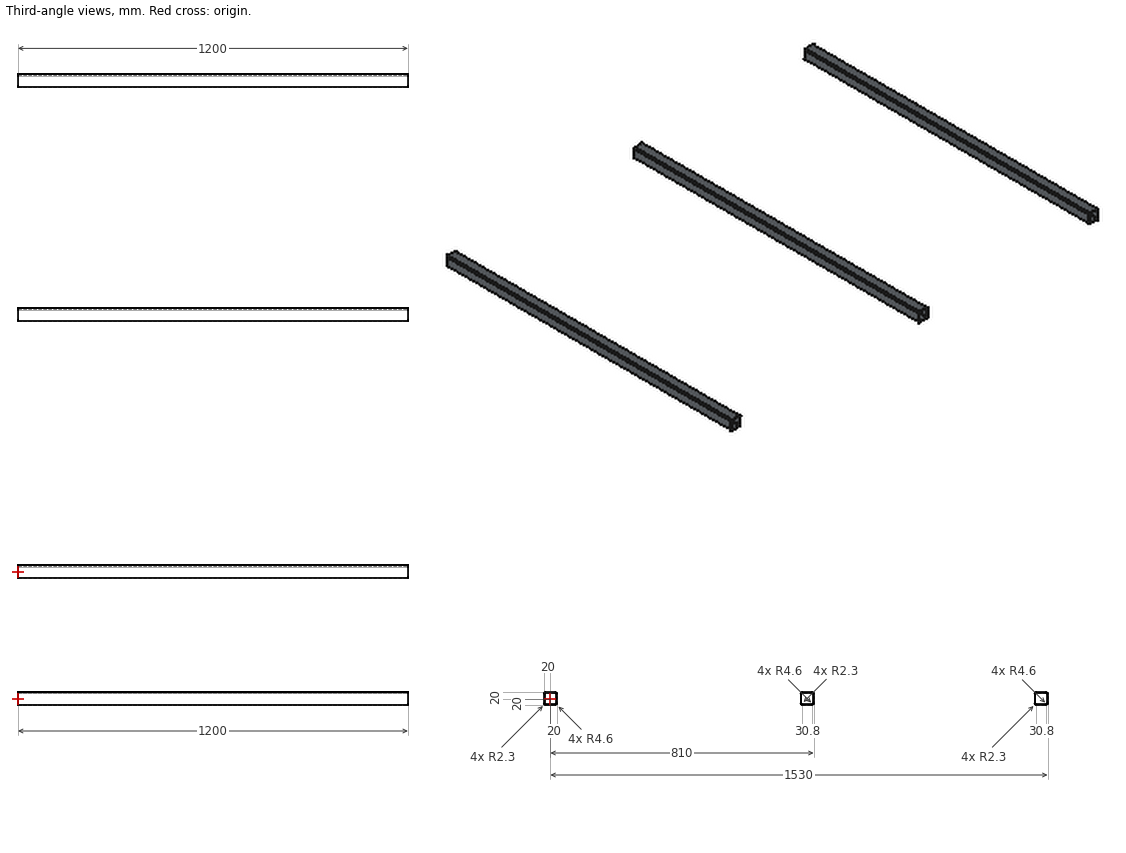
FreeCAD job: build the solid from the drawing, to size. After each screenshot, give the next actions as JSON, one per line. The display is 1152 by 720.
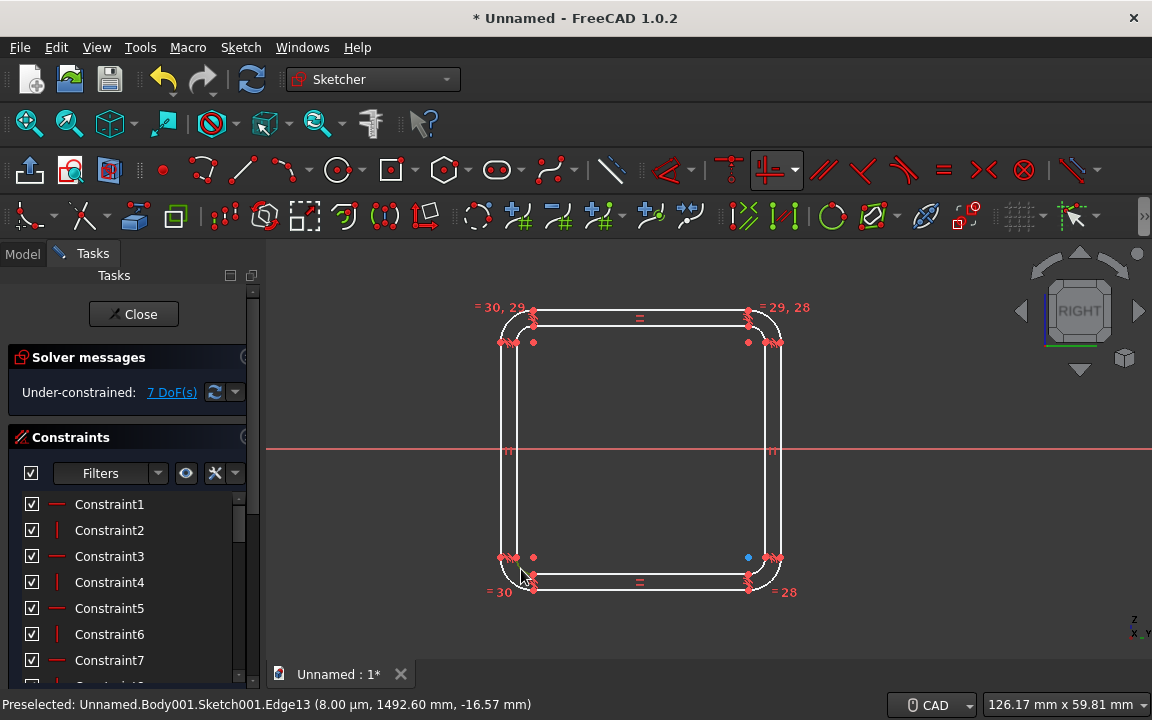
{"action": "left_click", "coordinate": [760, 569]}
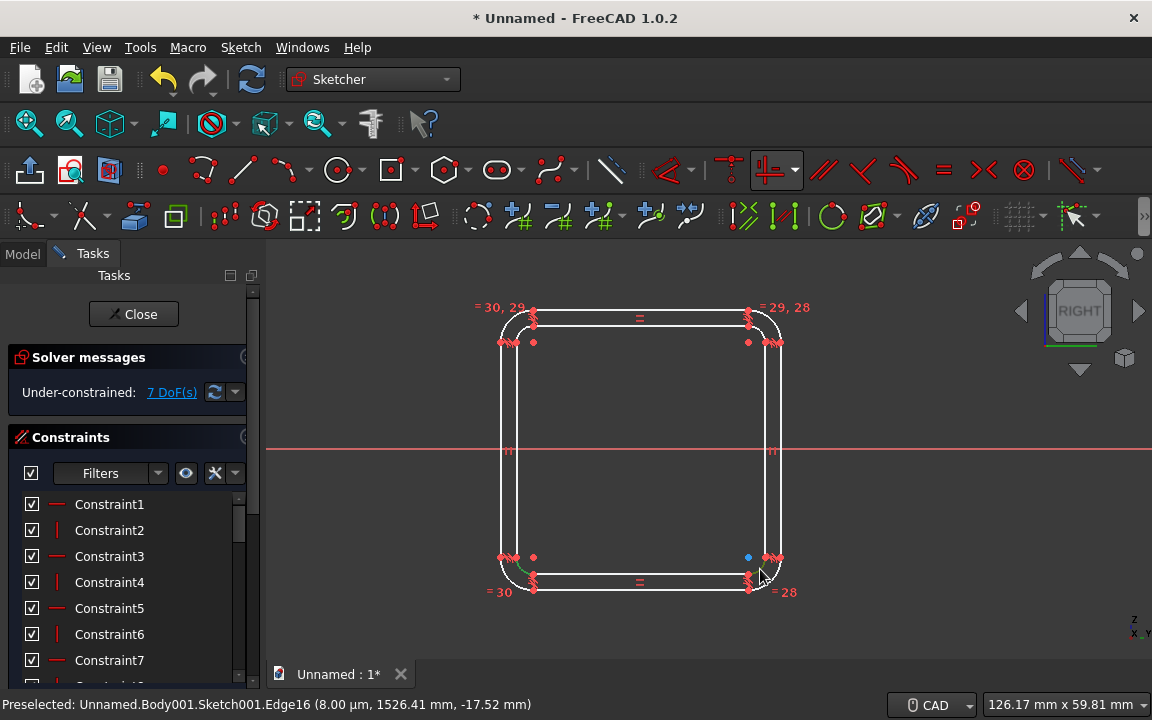
{"action": "key", "text": "e"}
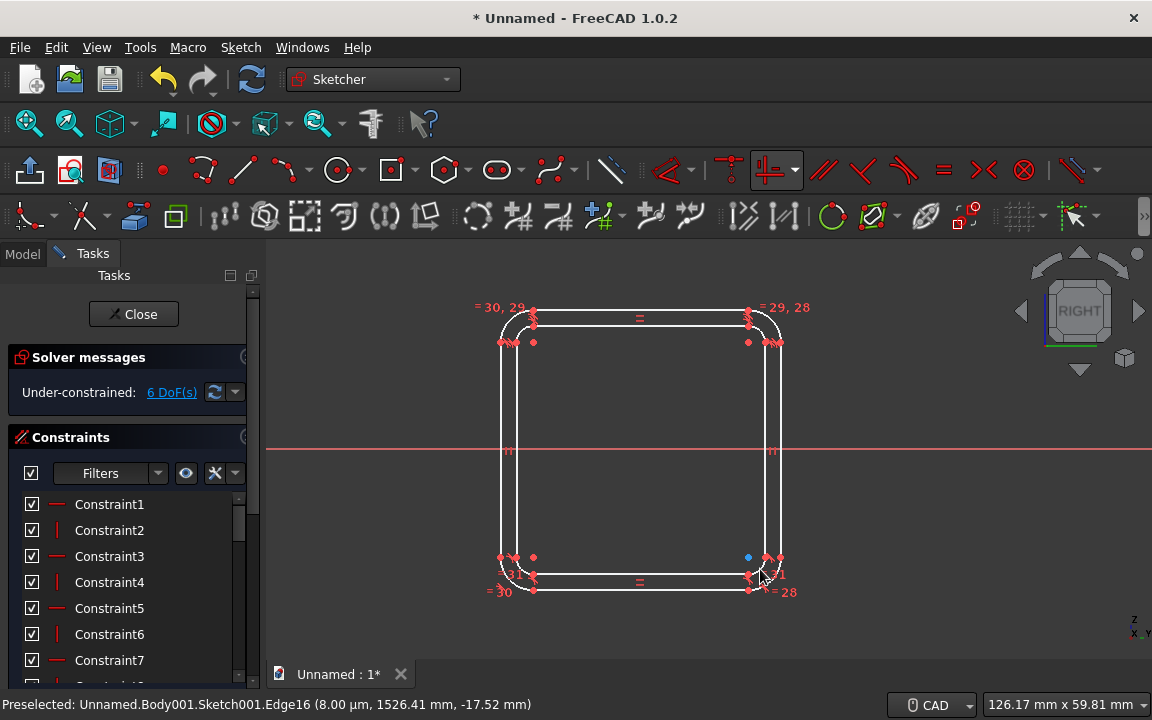
{"action": "left_click", "coordinate": [666, 170]}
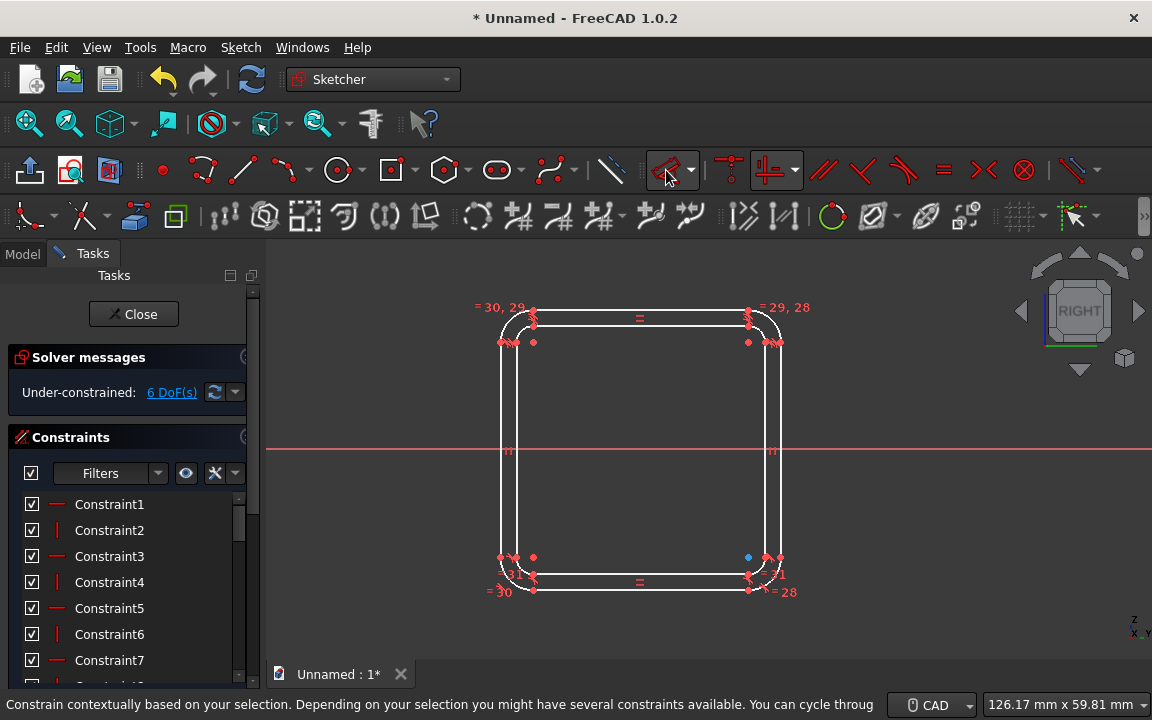
{"action": "scroll", "coordinate": [763, 587], "scroll_direction": "up", "scroll_amount": 2}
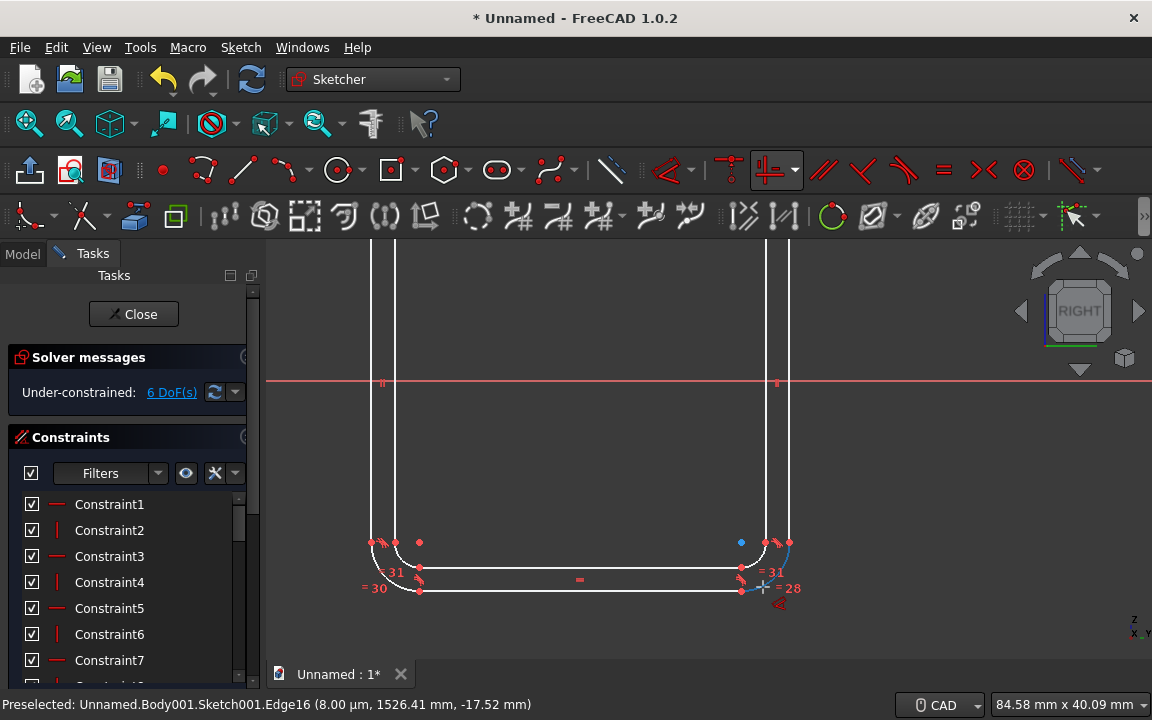
{"action": "left_click", "coordinate": [763, 586]}
{"action": "left_click", "coordinate": [777, 615]}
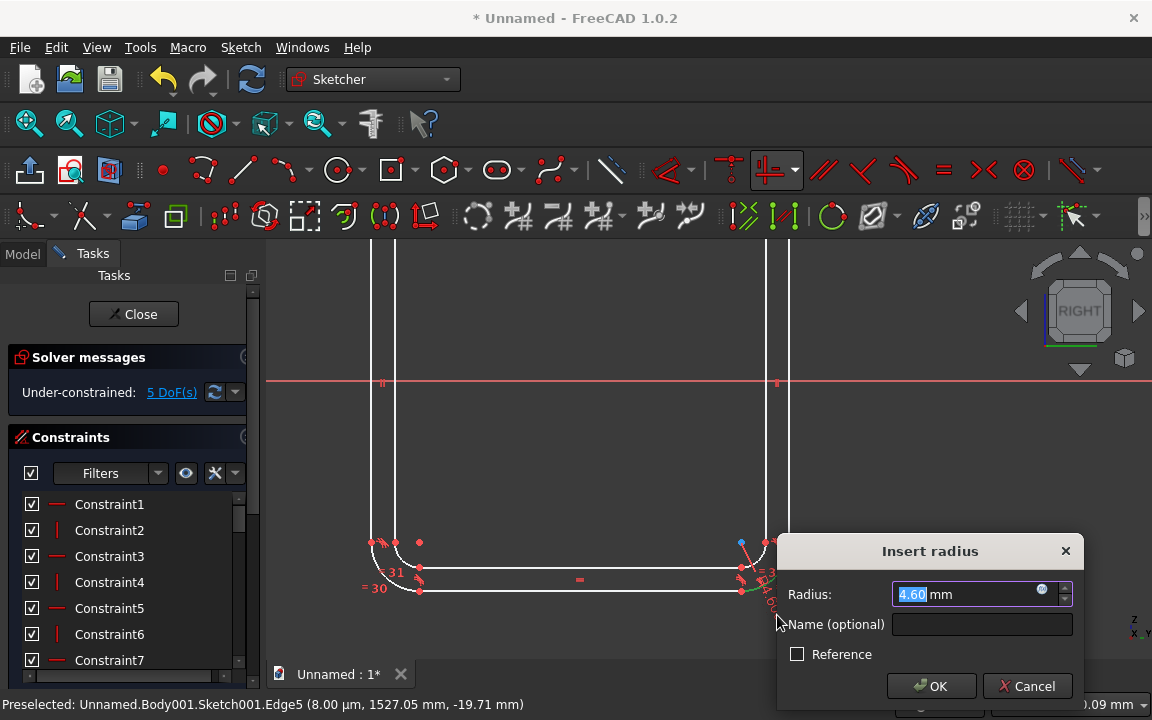
{"action": "type", "text": "4.6"}
{"action": "key", "text": "Return"}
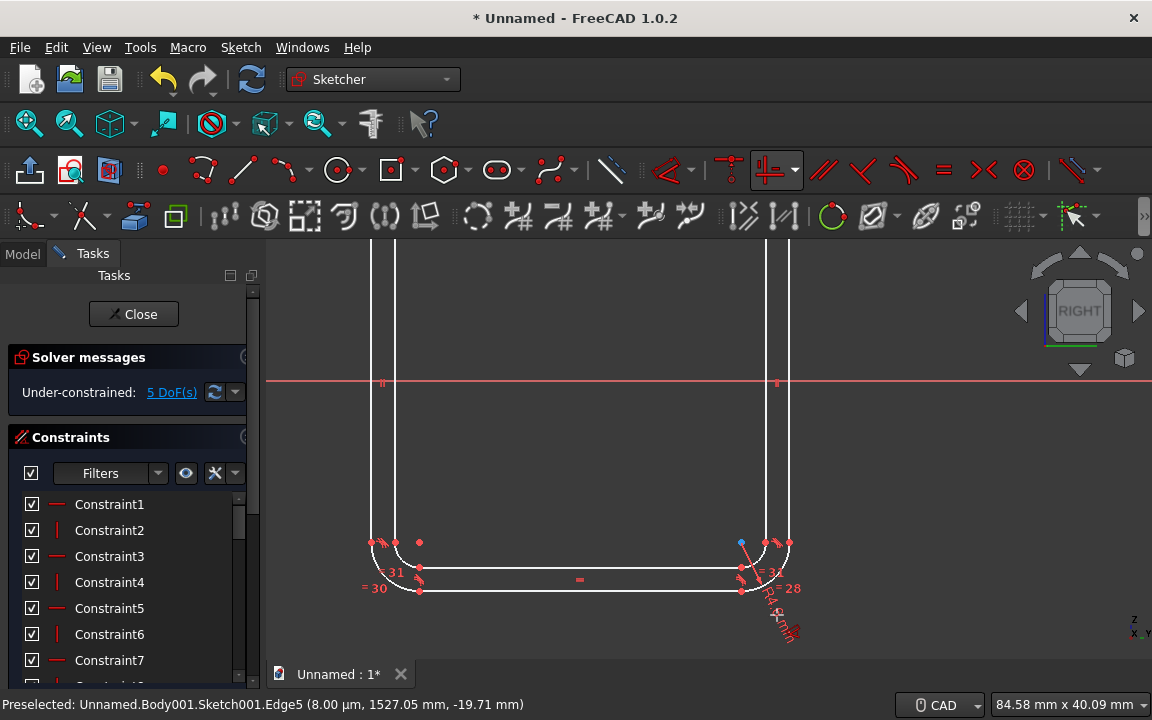
{"action": "scroll", "coordinate": [398, 554], "scroll_direction": "up", "scroll_amount": 3}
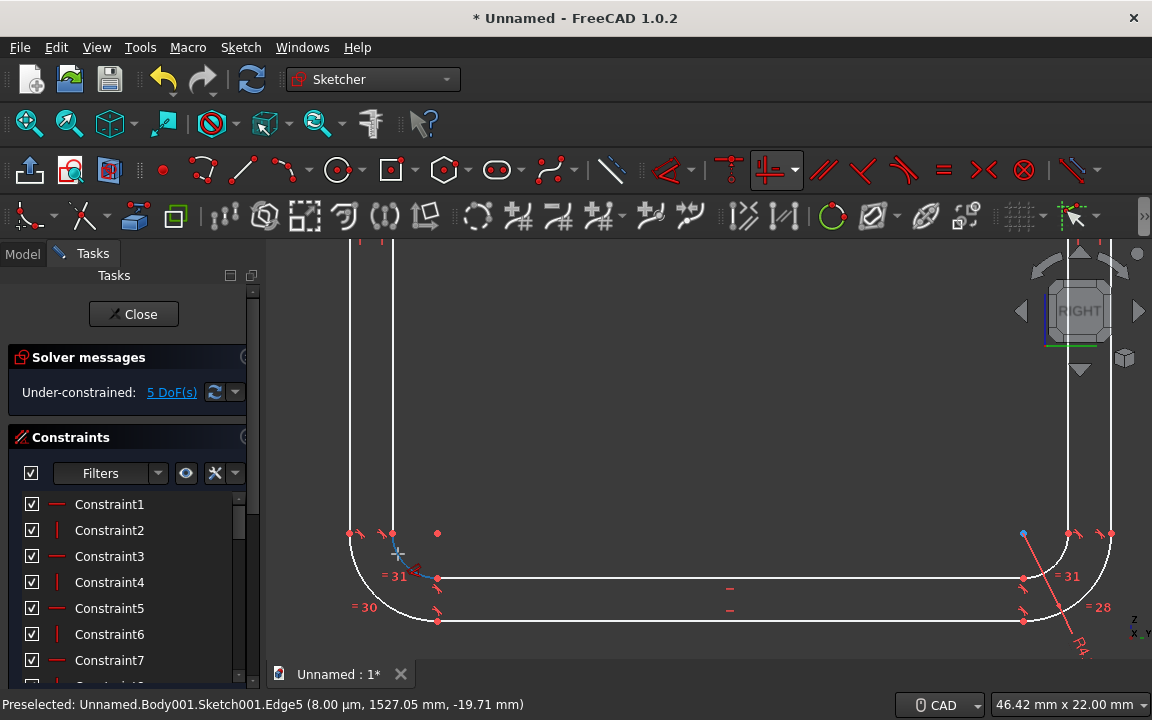
{"action": "left_click", "coordinate": [397, 554]}
{"action": "left_click", "coordinate": [370, 494]}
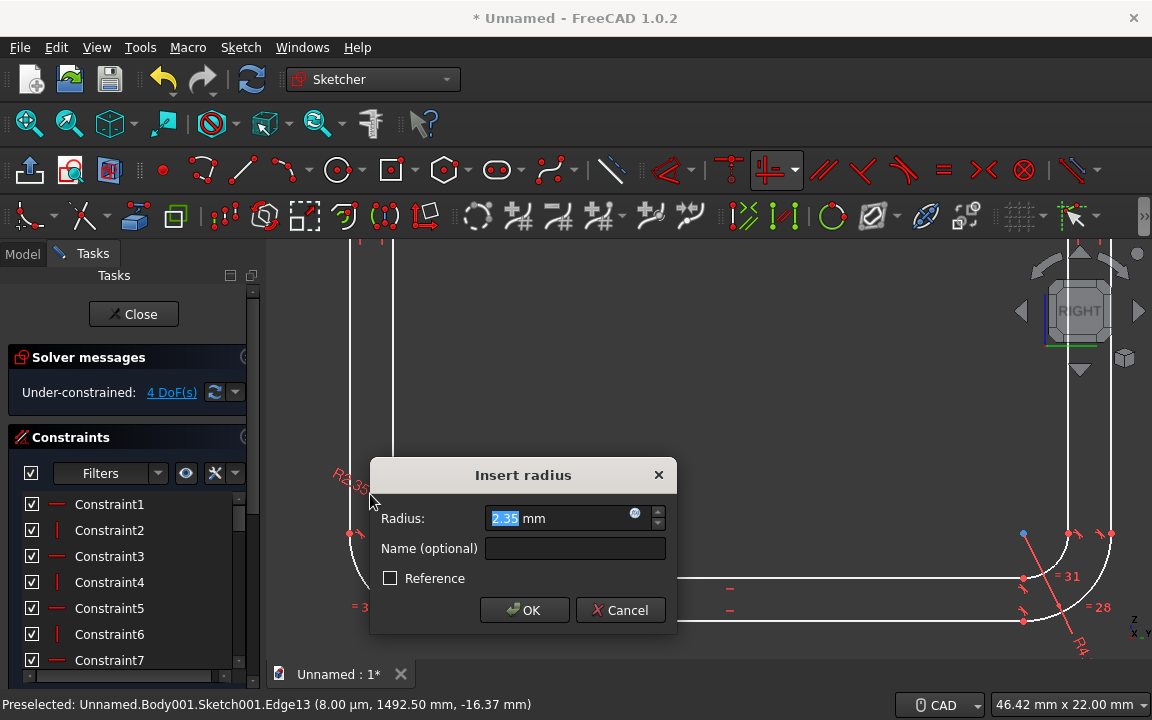
{"action": "type", "text": "2.3"}
{"action": "key", "text": "Return"}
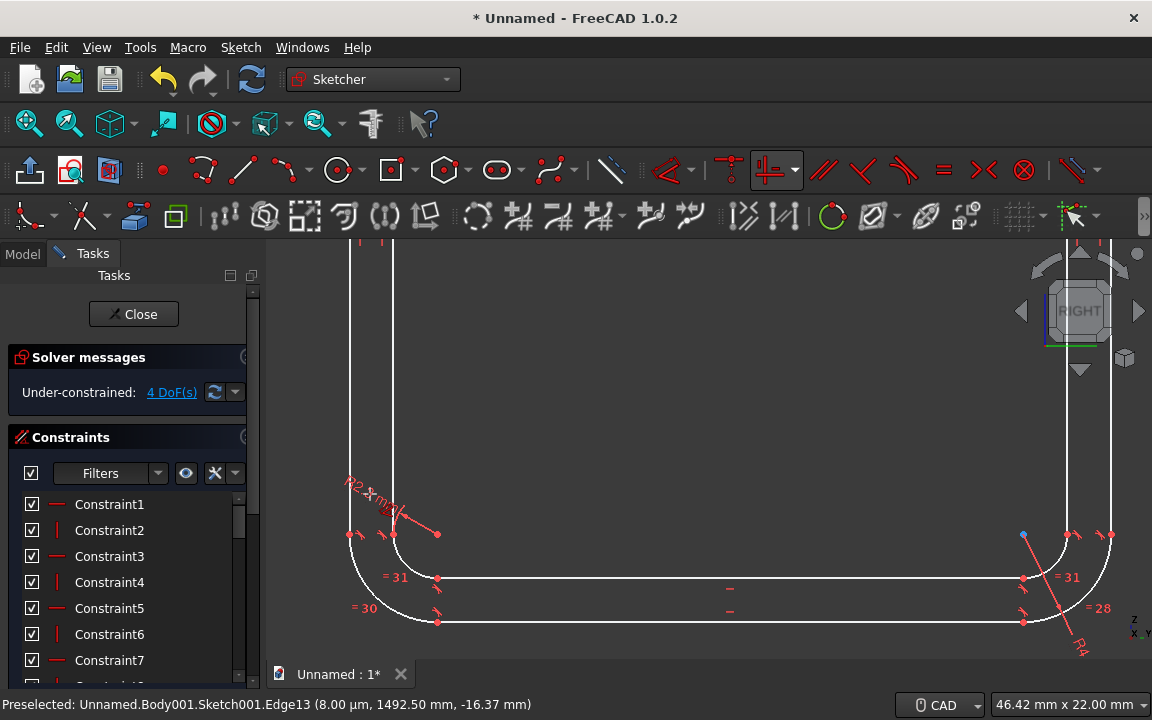
{"action": "left_click", "coordinate": [437, 622]}
{"action": "left_click", "coordinate": [471, 445]}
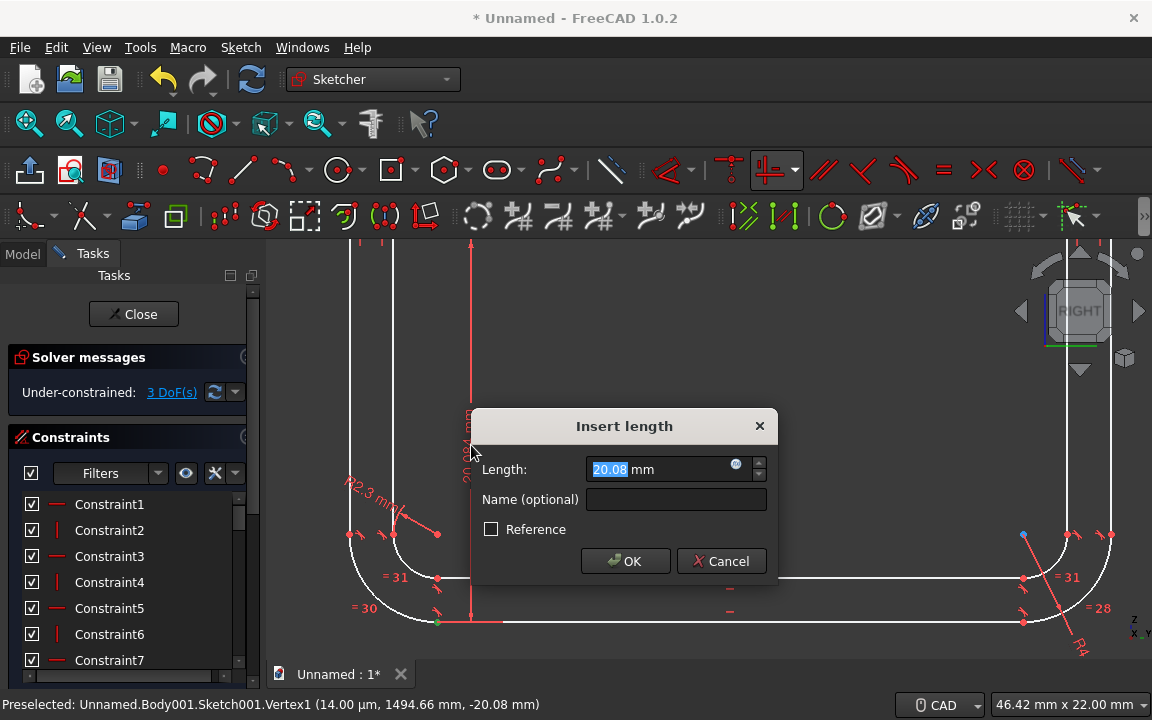
{"action": "type", "text": "20"}
{"action": "key", "text": "Return"}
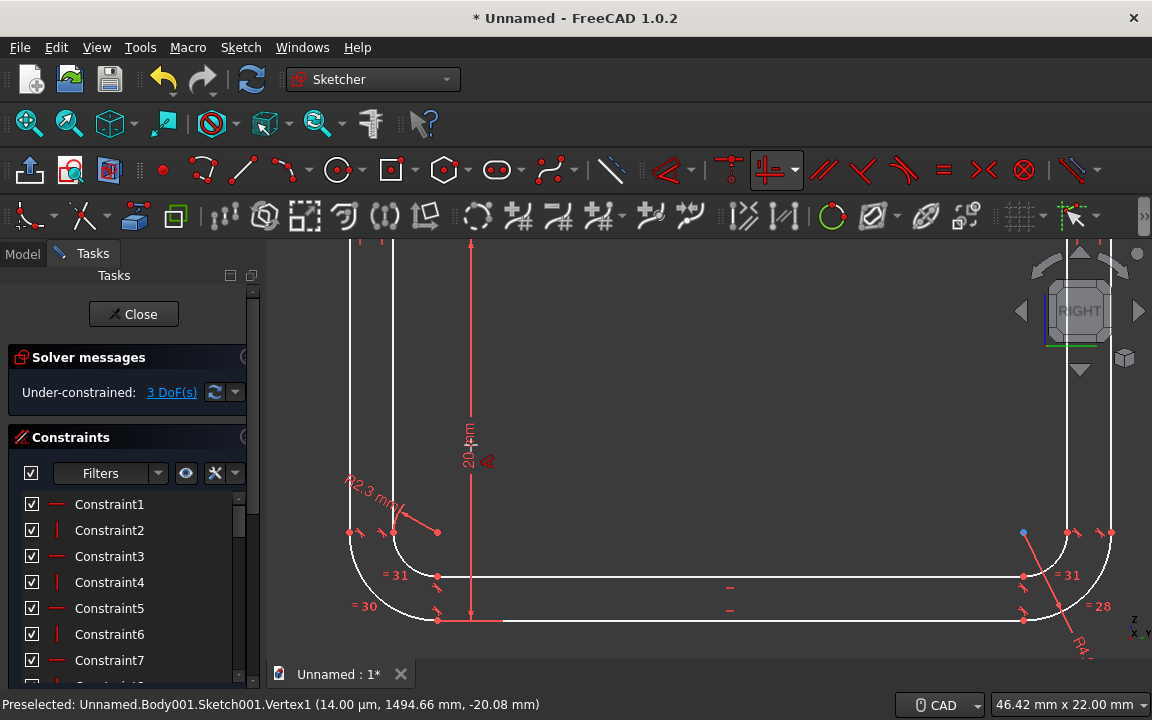
{"action": "scroll", "coordinate": [588, 571], "scroll_direction": "down", "scroll_amount": 5}